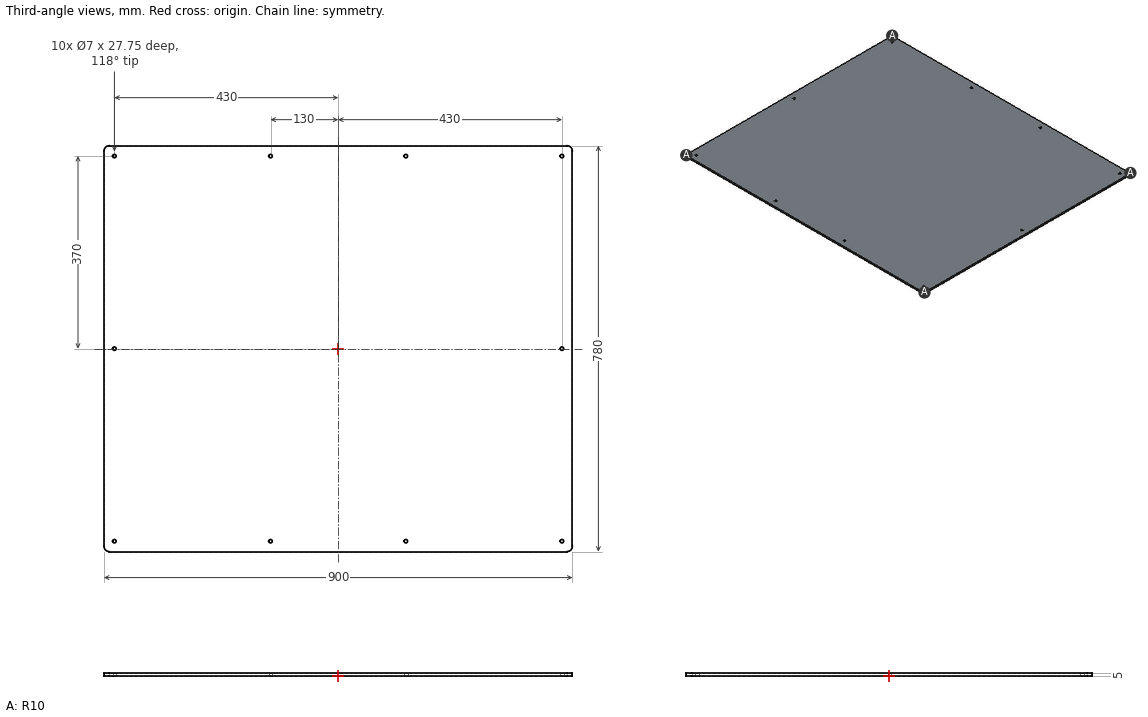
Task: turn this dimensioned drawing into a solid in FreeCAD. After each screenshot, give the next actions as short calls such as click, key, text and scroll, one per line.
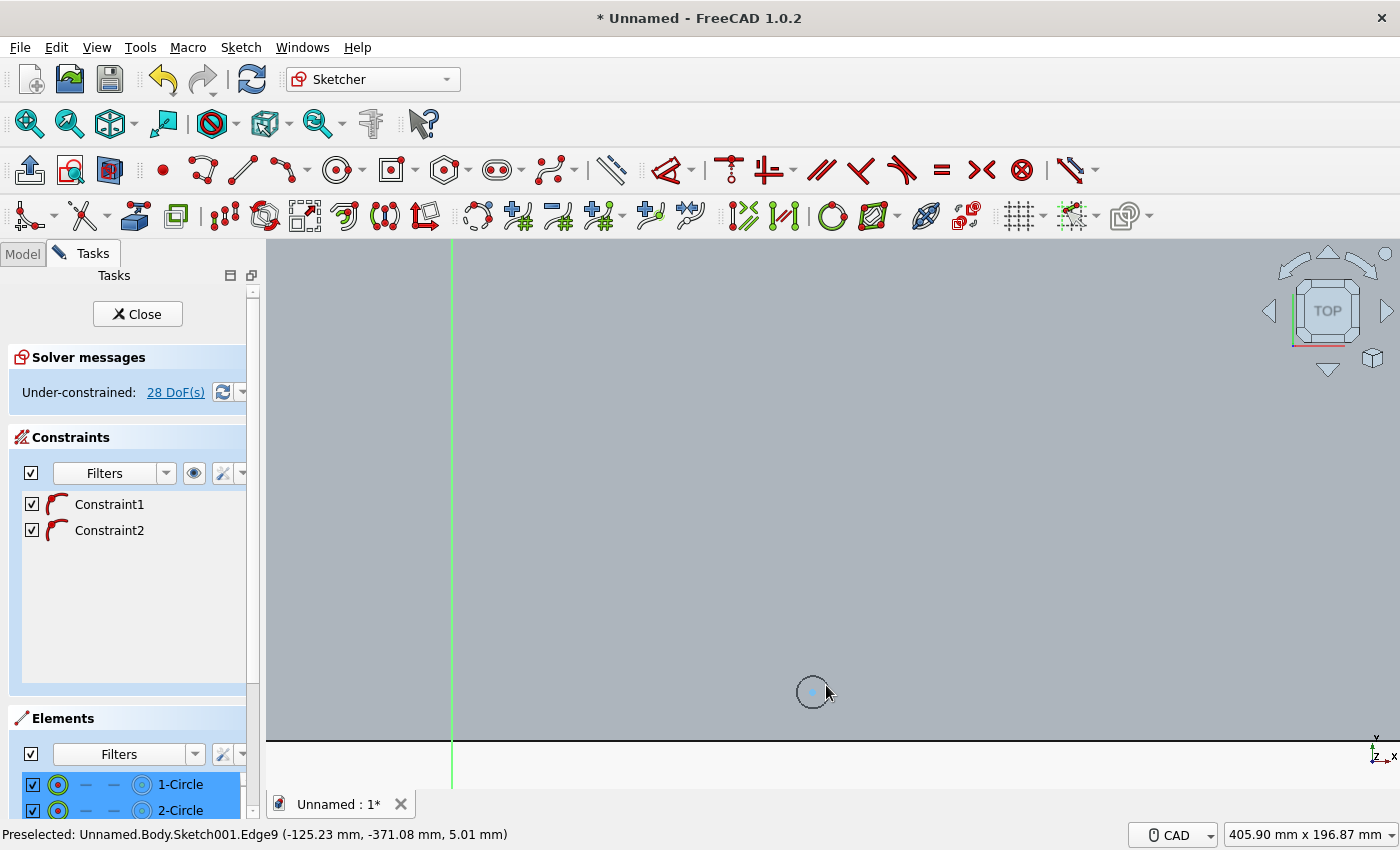
click(824, 681)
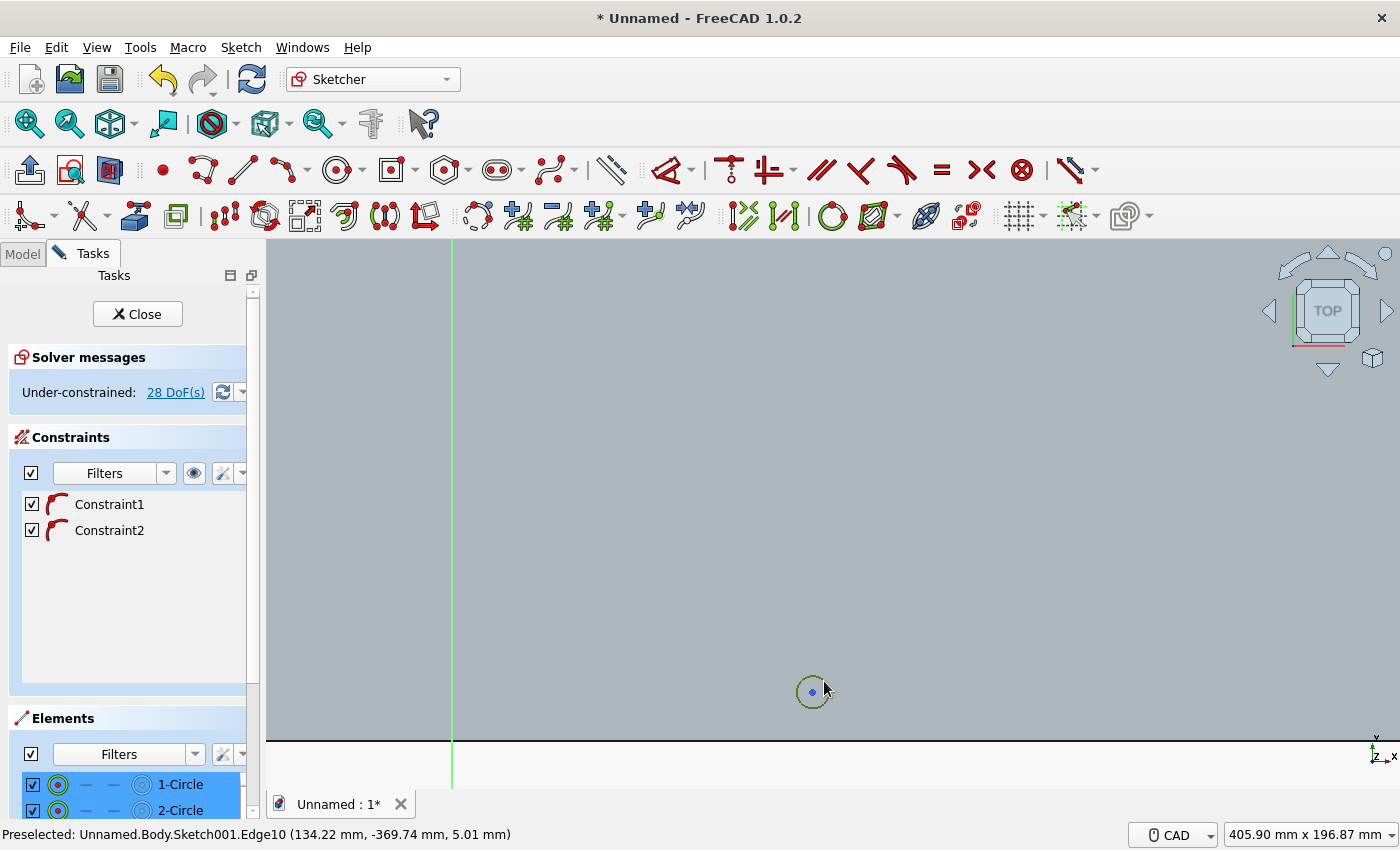
click(942, 170)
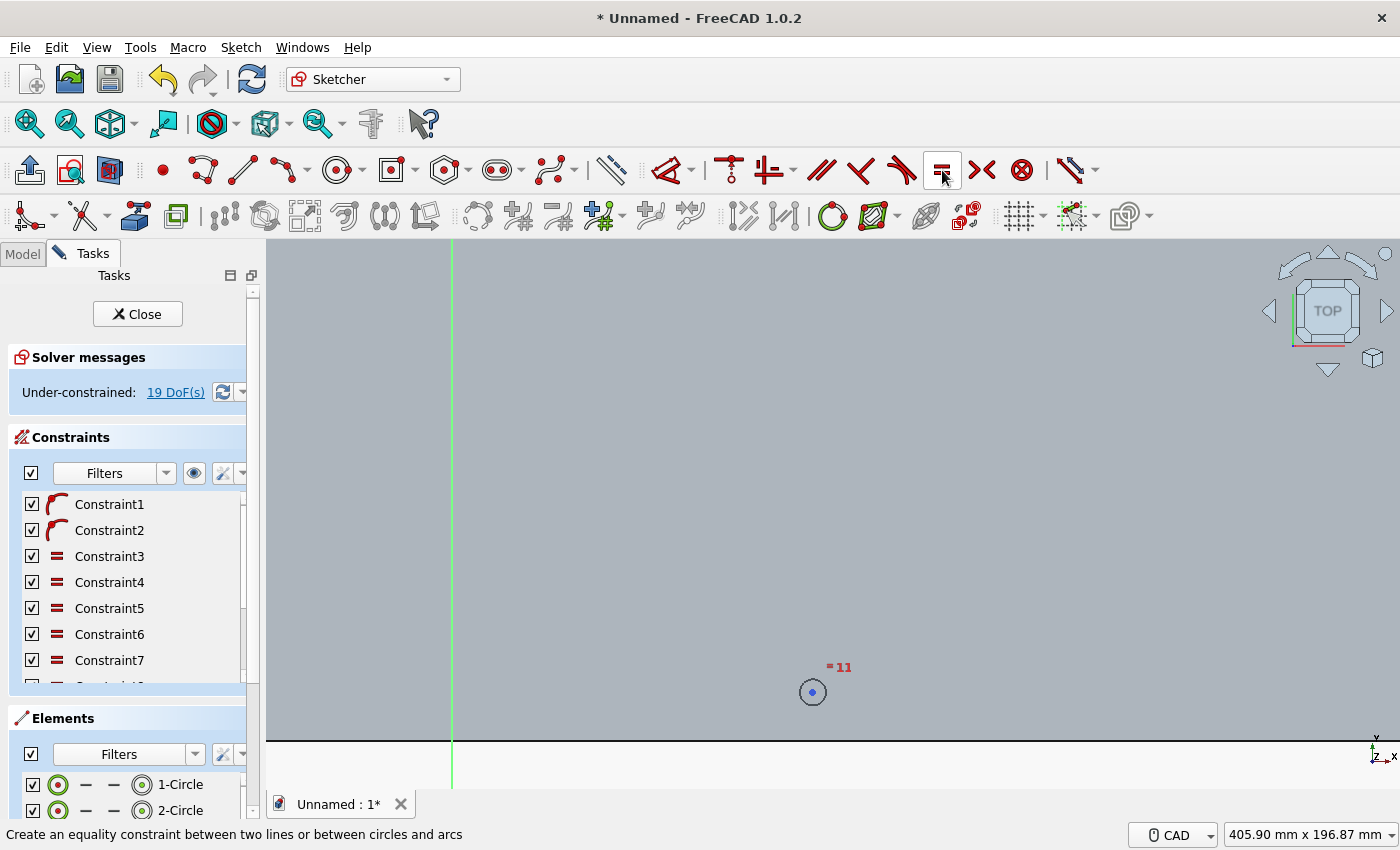
scroll(826, 685, down, 9)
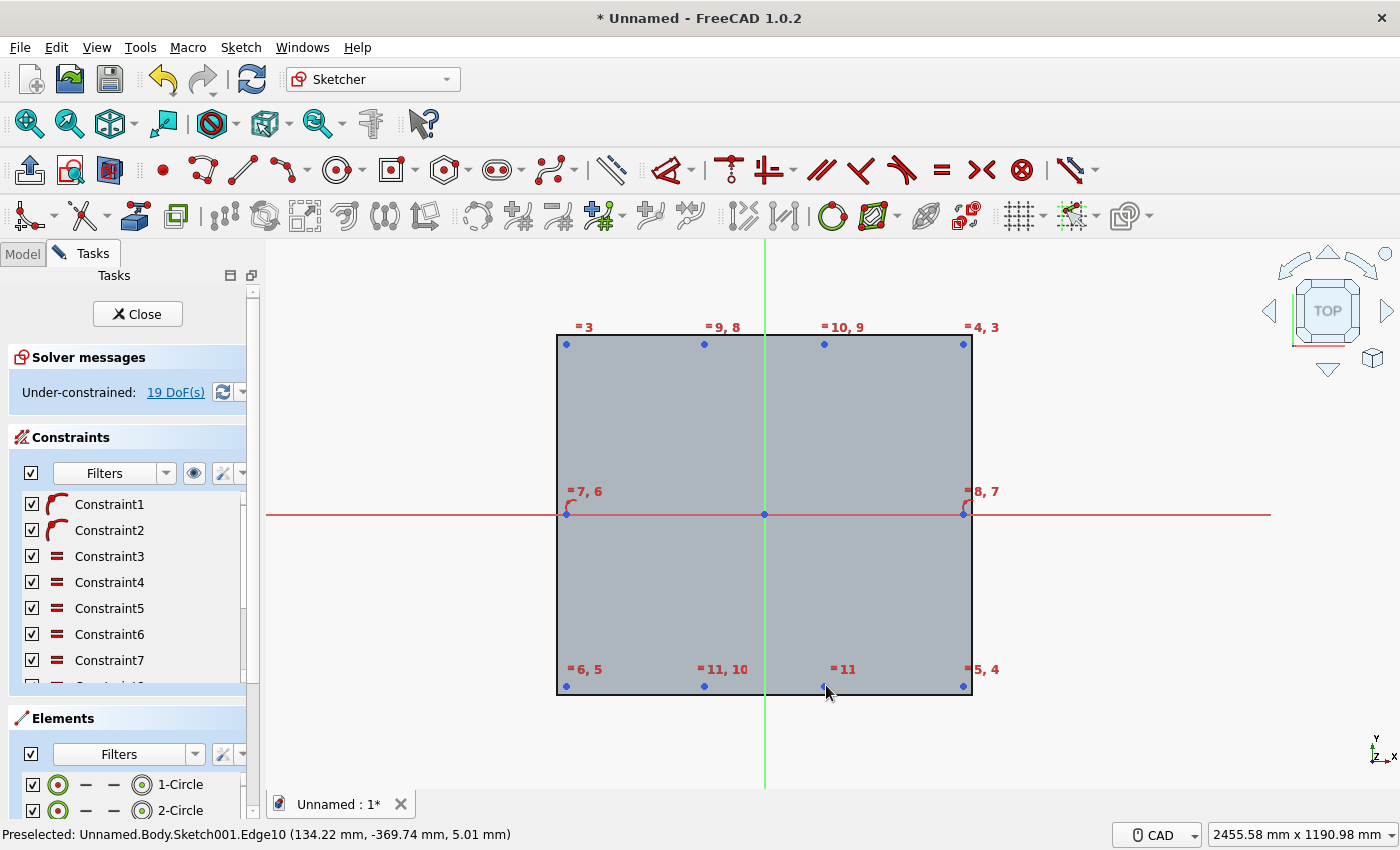
click(566, 345)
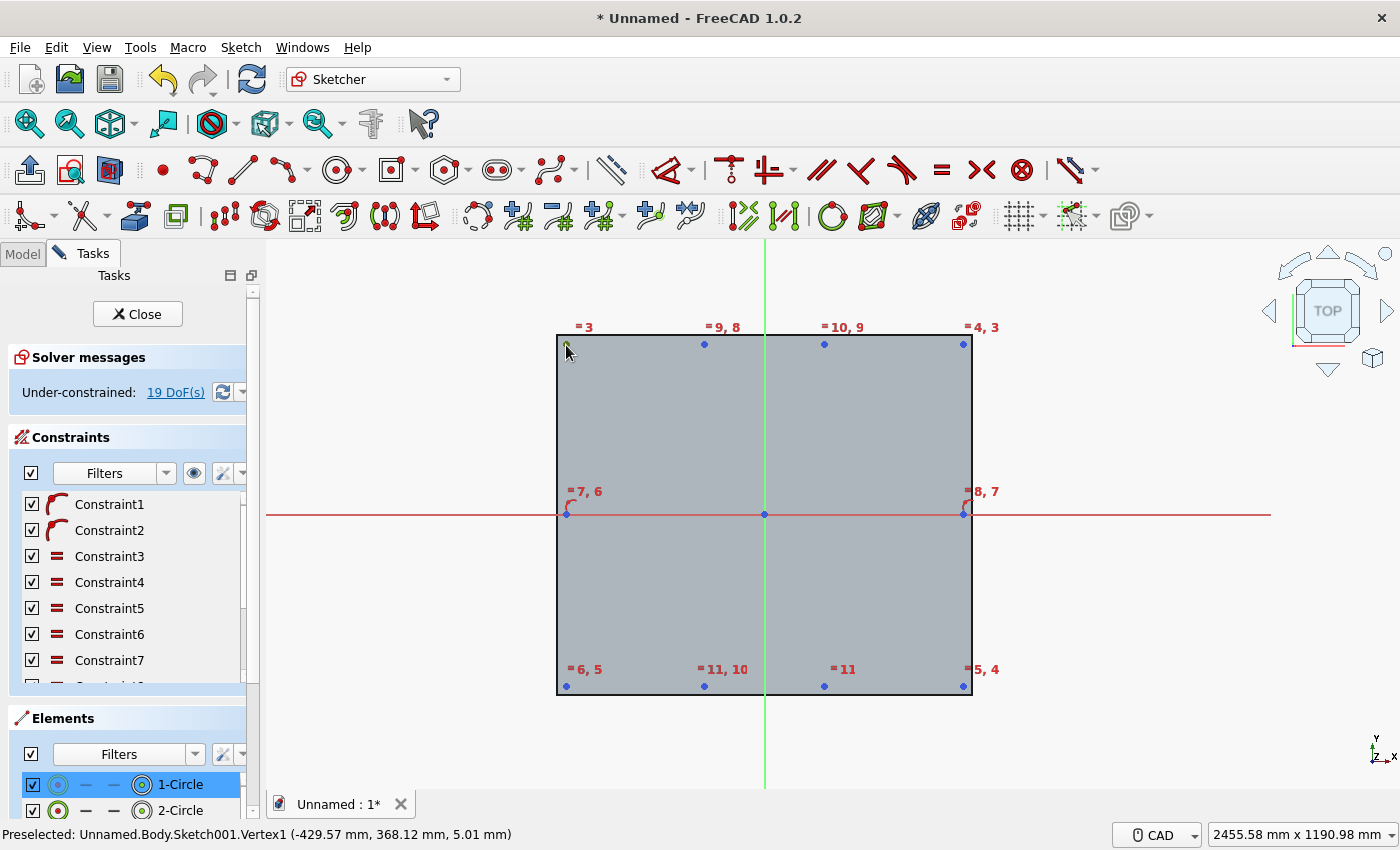
click(963, 345)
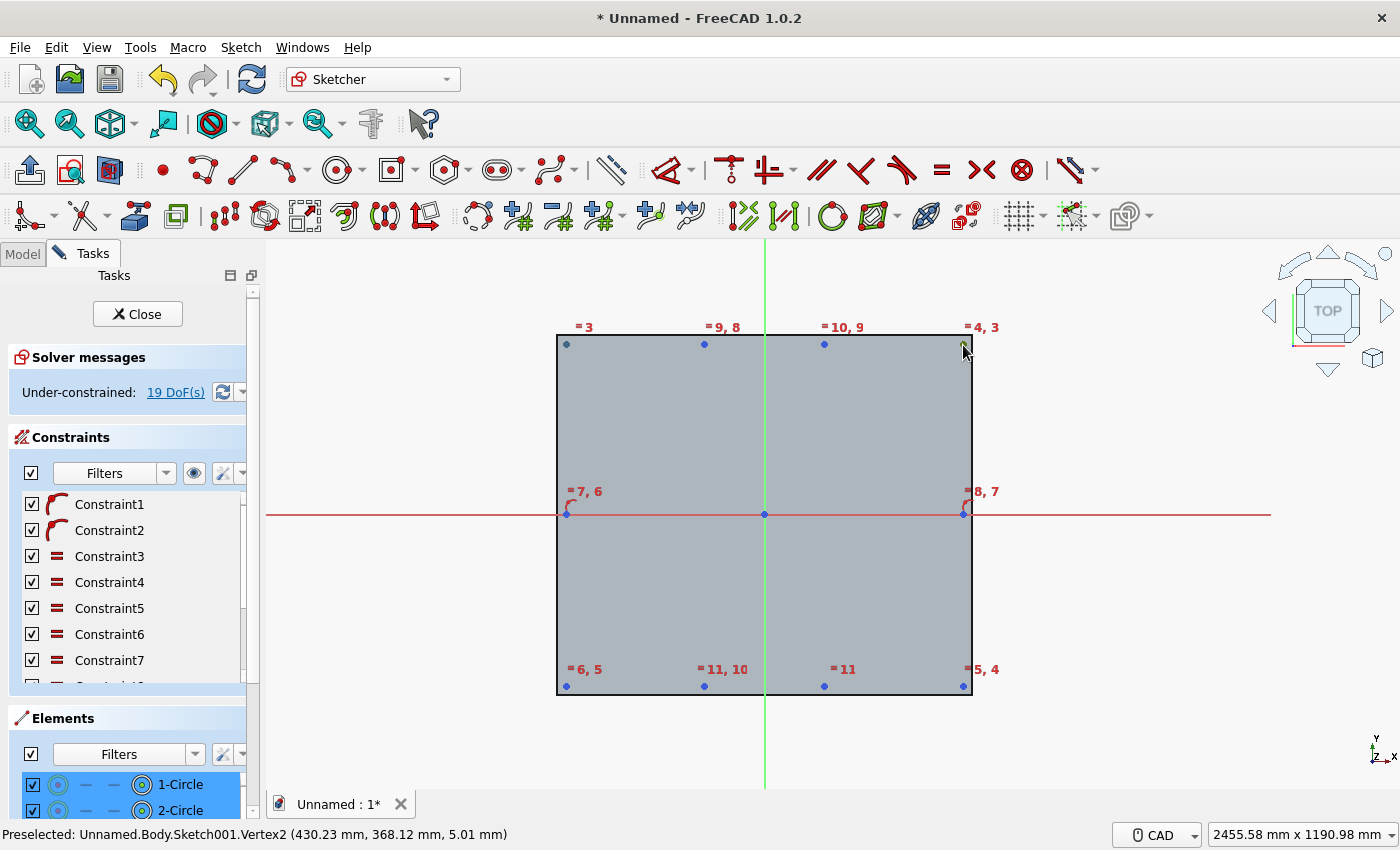
click(765, 726)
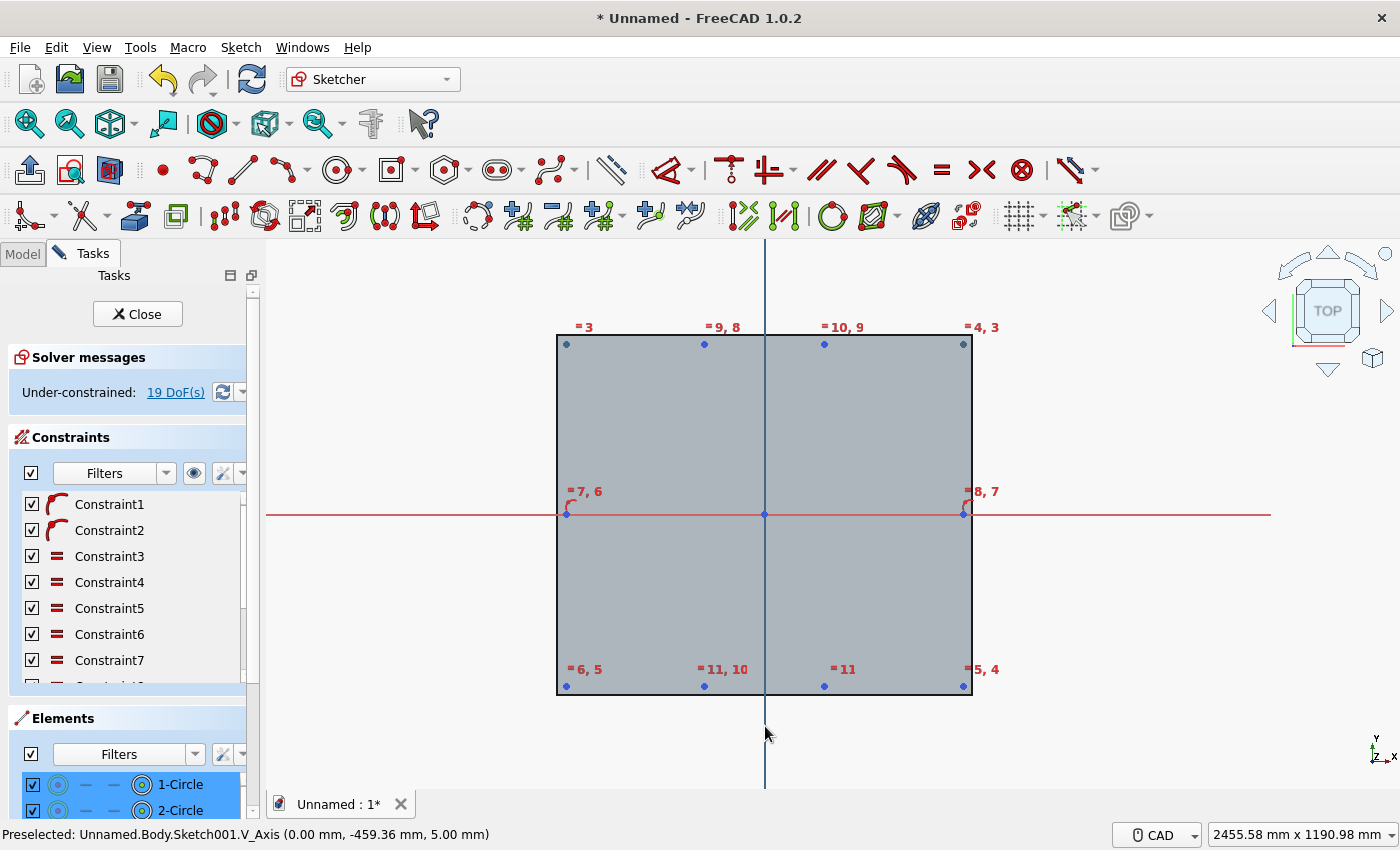
click(982, 170)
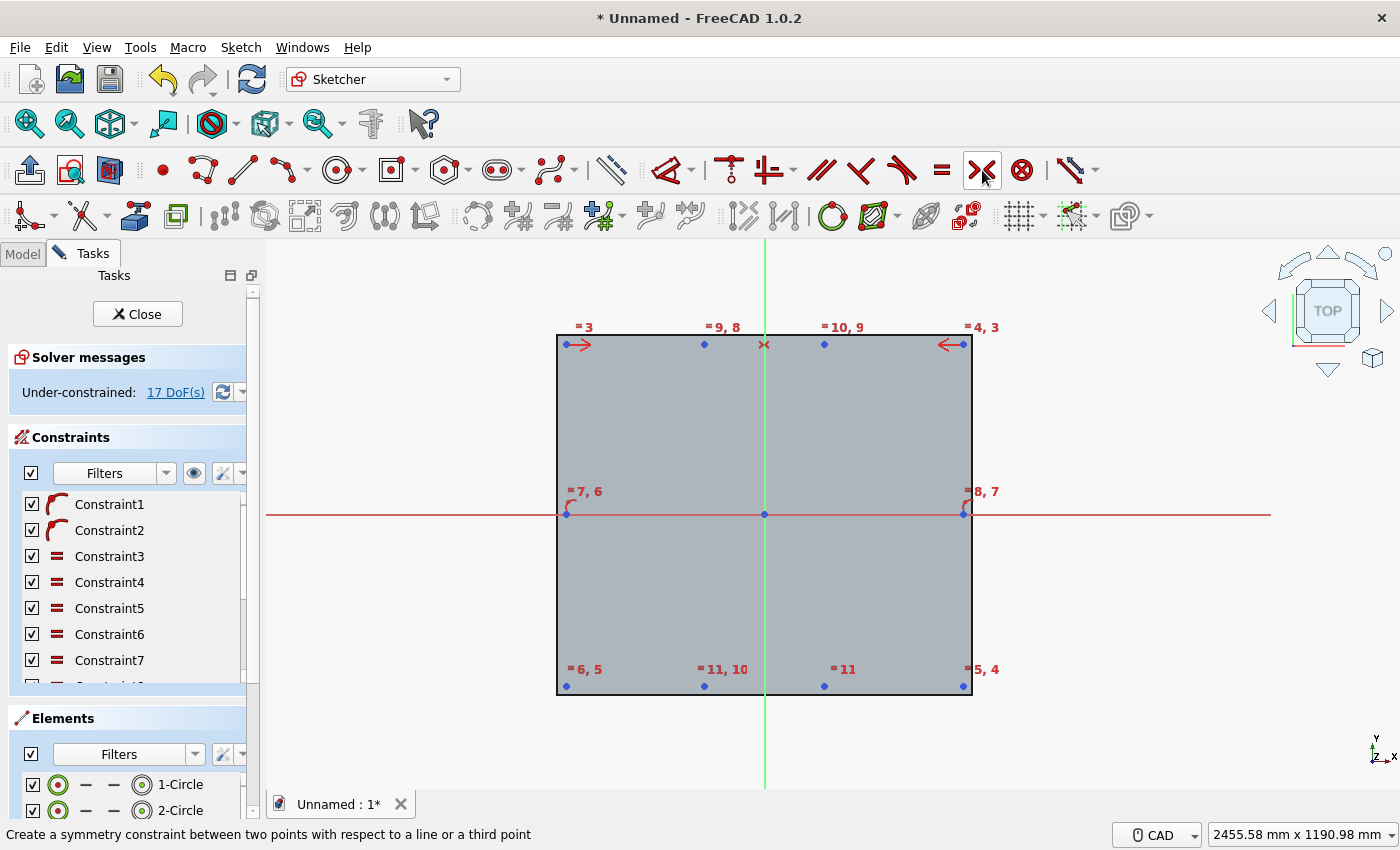
click(963, 345)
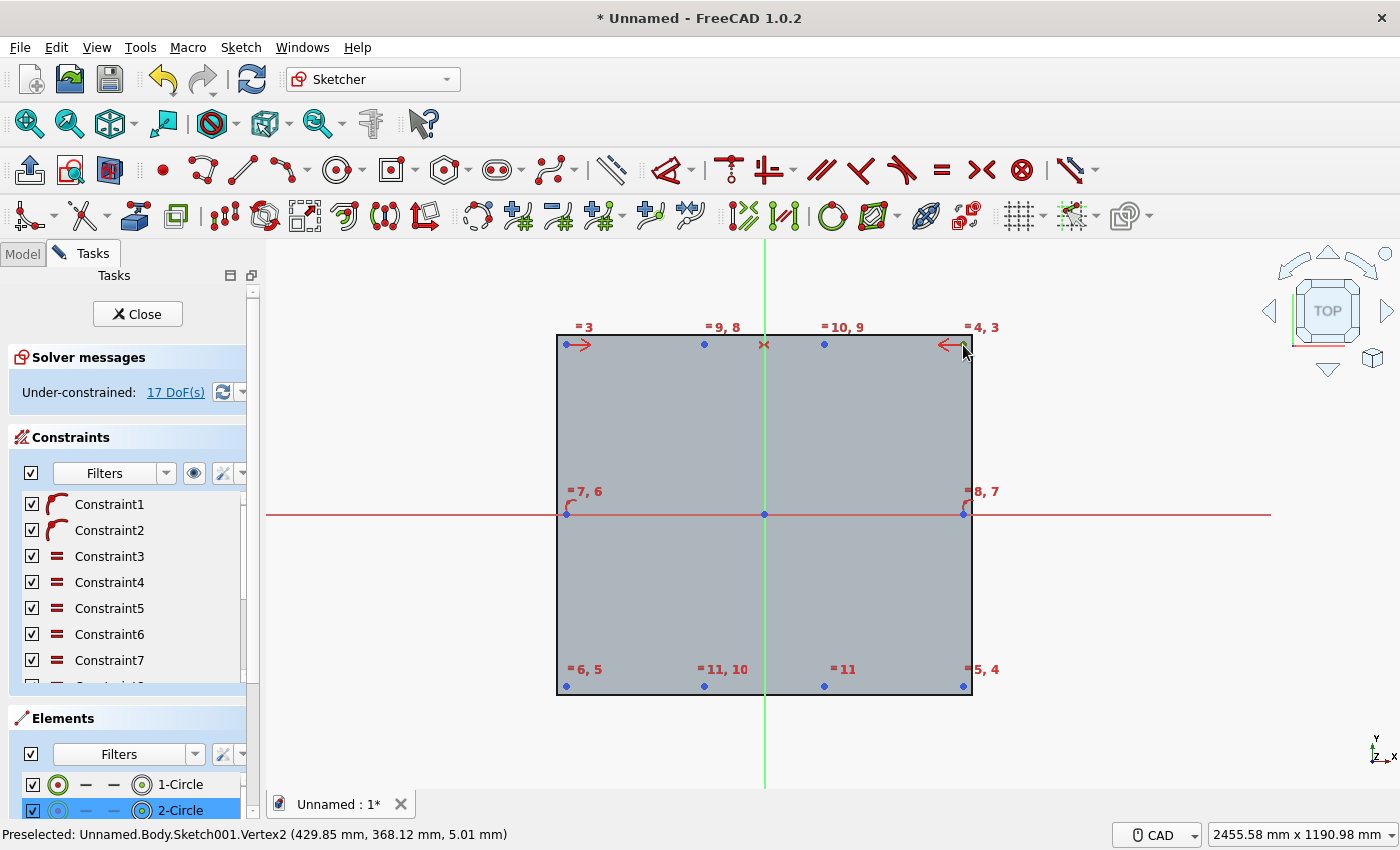
click(963, 687)